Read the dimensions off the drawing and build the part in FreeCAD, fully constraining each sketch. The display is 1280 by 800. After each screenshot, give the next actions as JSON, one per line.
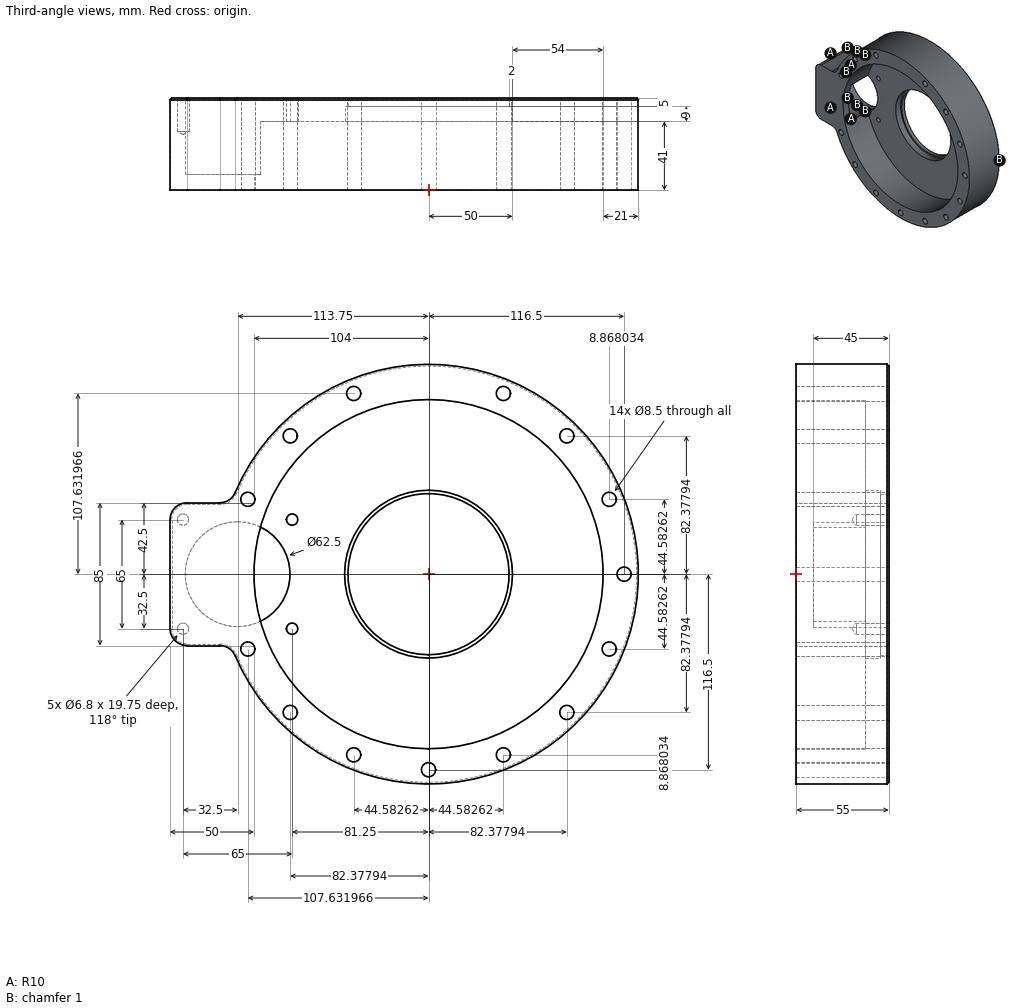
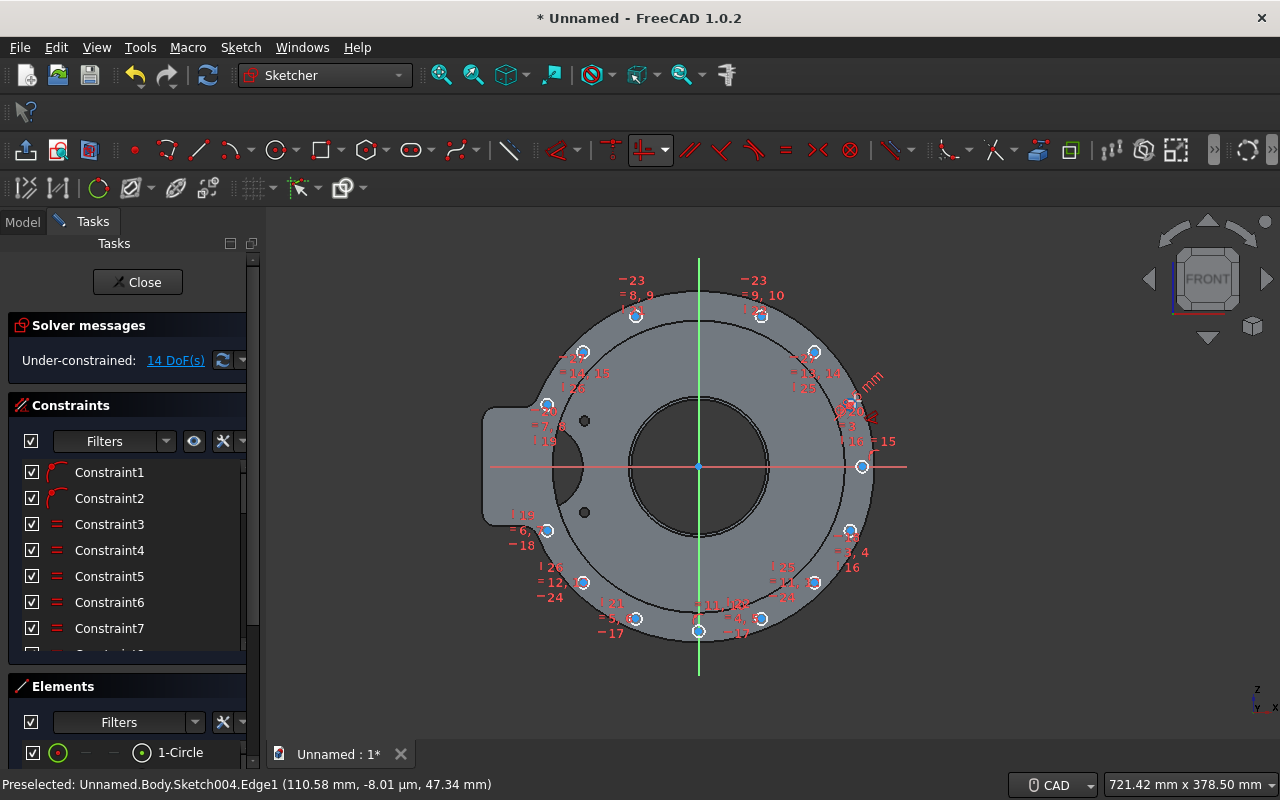
{"action": "left_click", "coordinate": [699, 631]}
{"action": "left_click", "coordinate": [665, 549]}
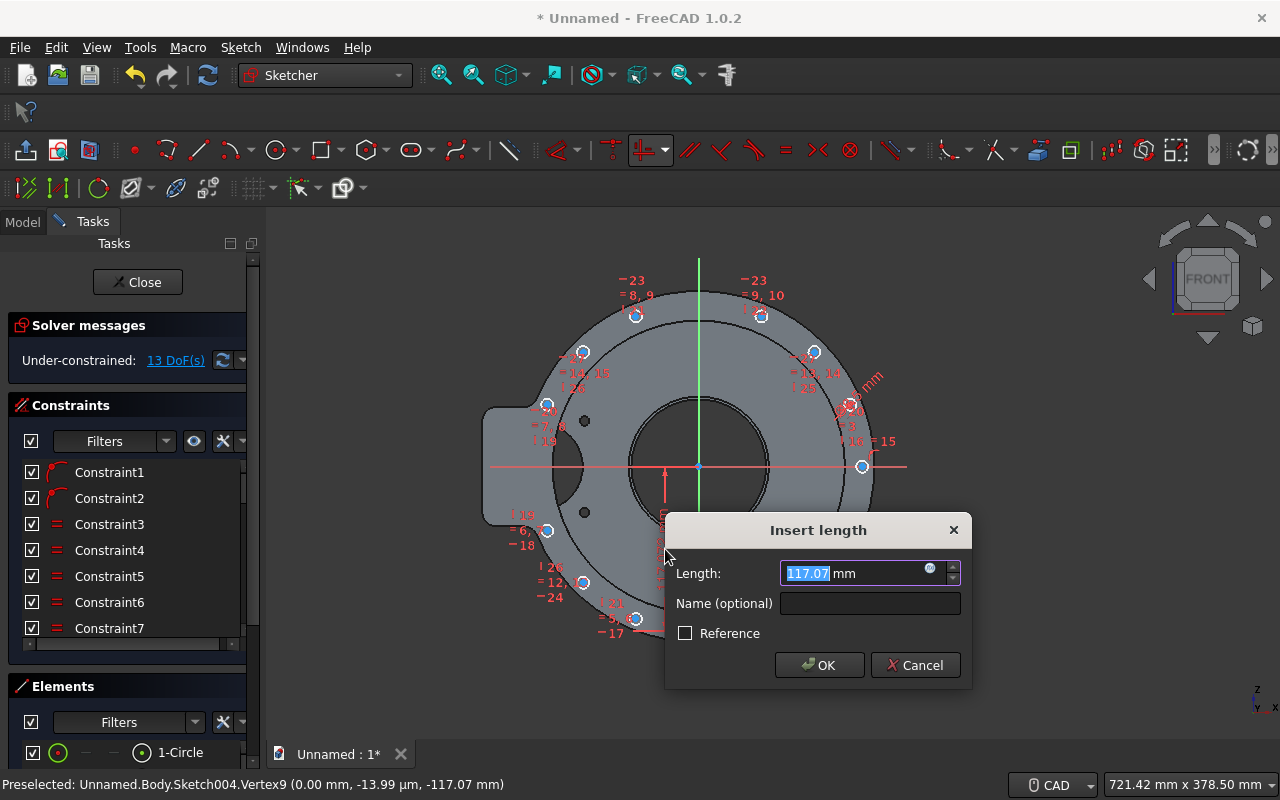
{"action": "type", "text": "116.5"}
{"action": "key", "text": "Return"}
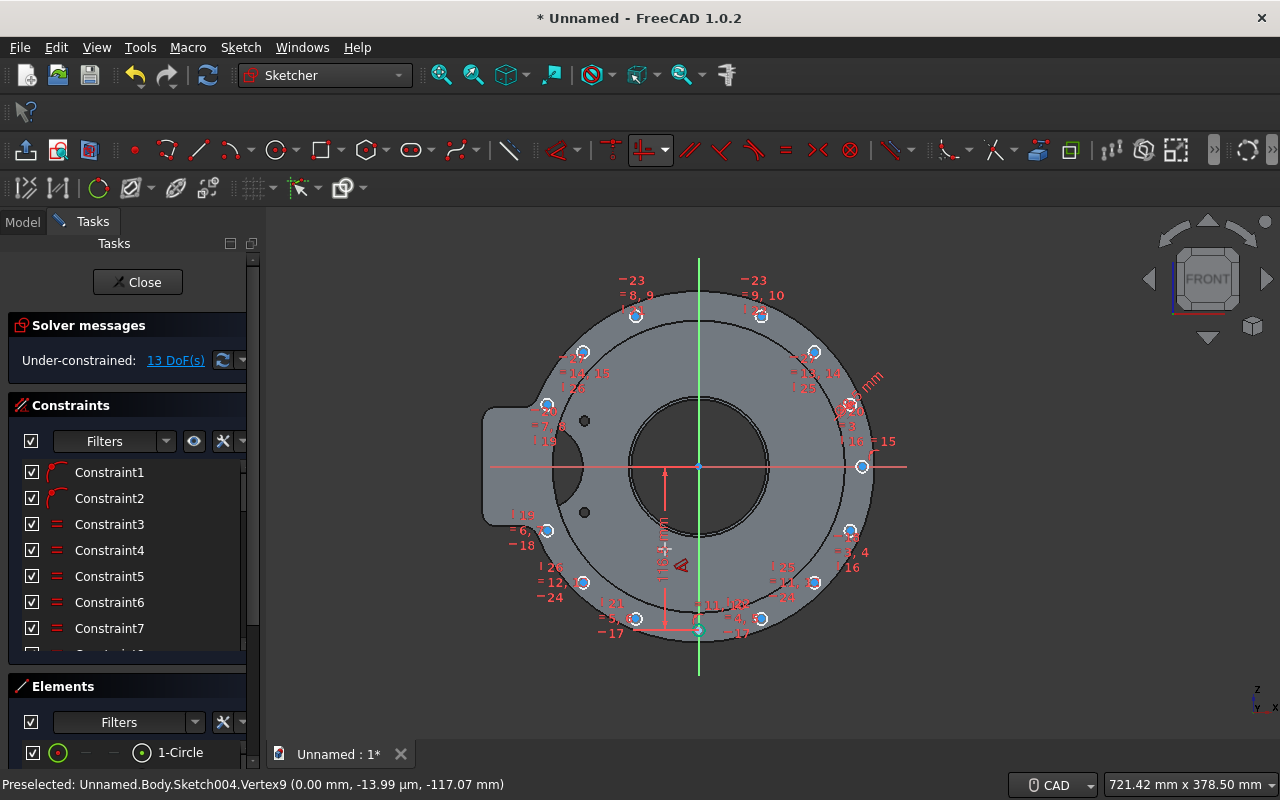
{"action": "left_click", "coordinate": [862, 467]}
{"action": "left_click", "coordinate": [780, 433]}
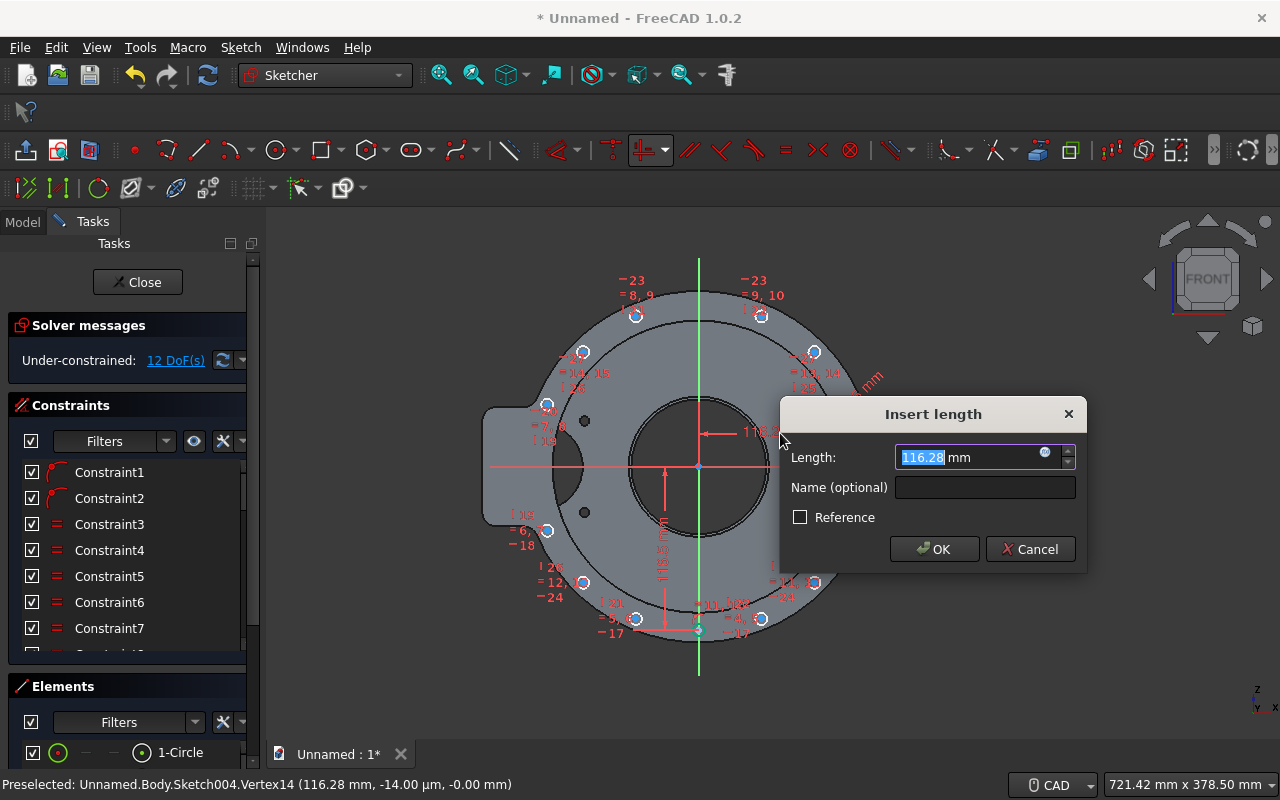
{"action": "type", "text": "116.5"}
{"action": "key", "text": "Return"}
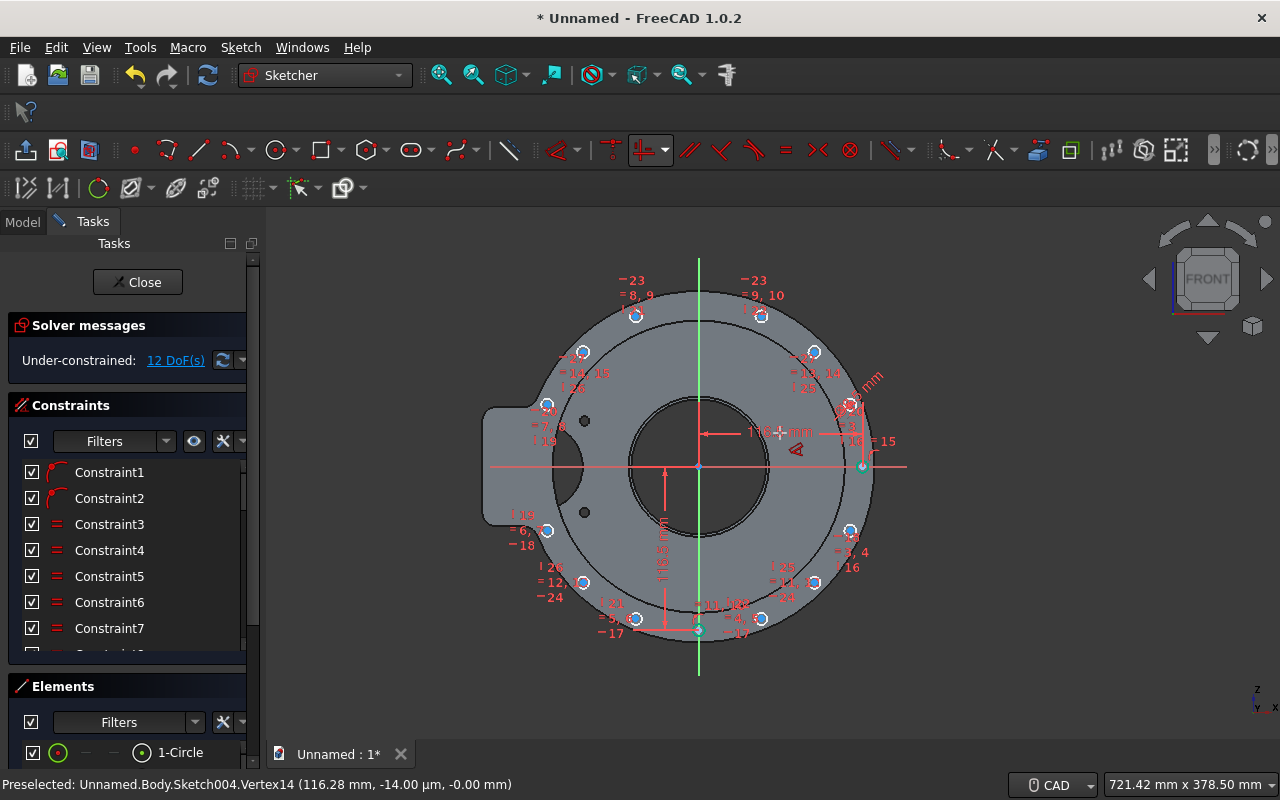
{"action": "left_click", "coordinate": [850, 405]}
{"action": "left_click", "coordinate": [884, 436]}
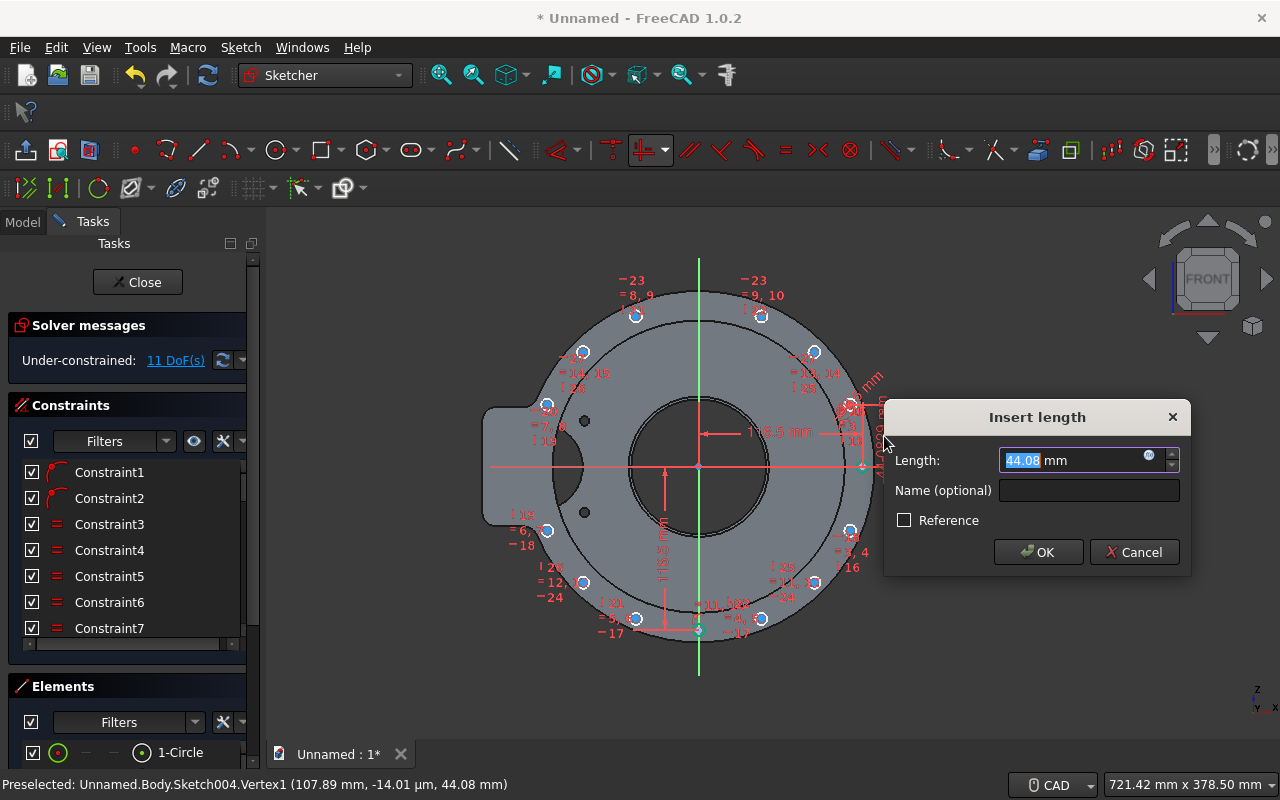
{"action": "type", "text": "44.58262"}
{"action": "key", "text": "Return"}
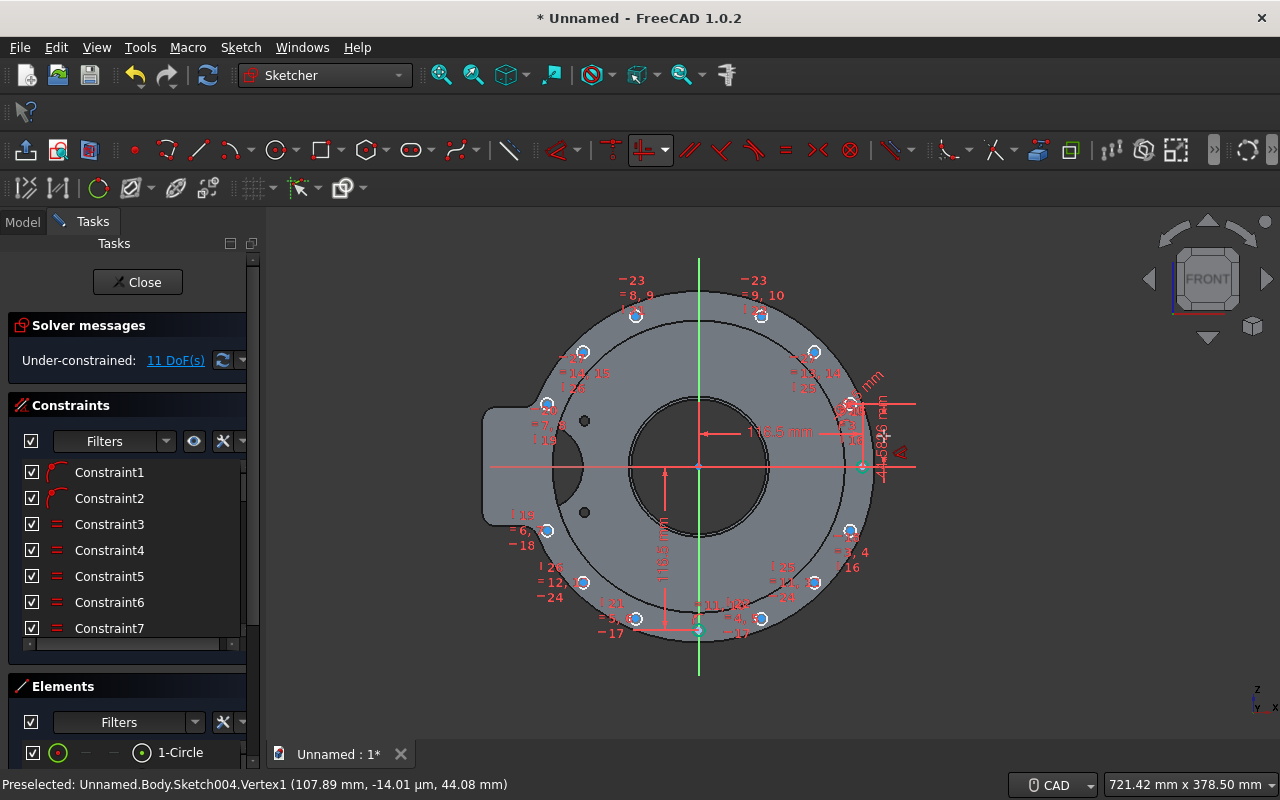
{"action": "left_click", "coordinate": [850, 531]}
{"action": "left_click", "coordinate": [884, 499]}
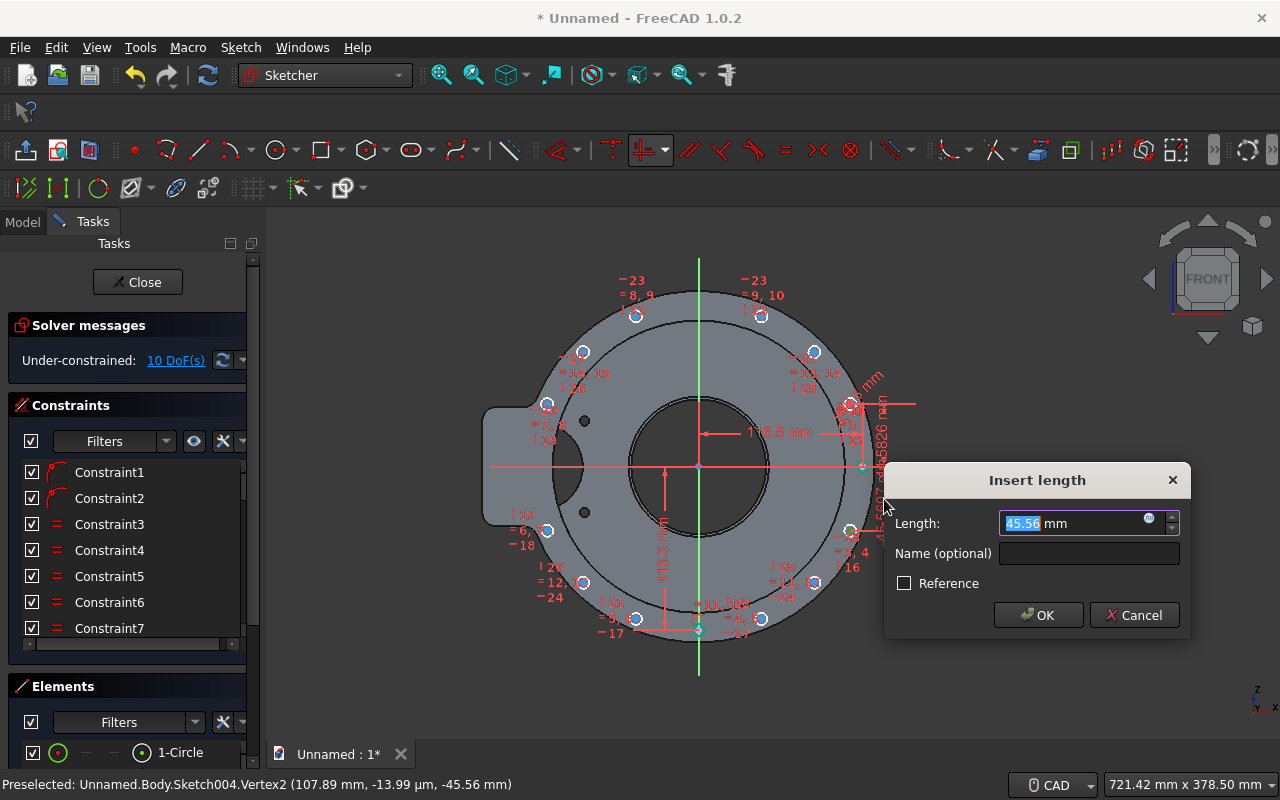
{"action": "type", "text": "44.58262"}
{"action": "key", "text": "Return"}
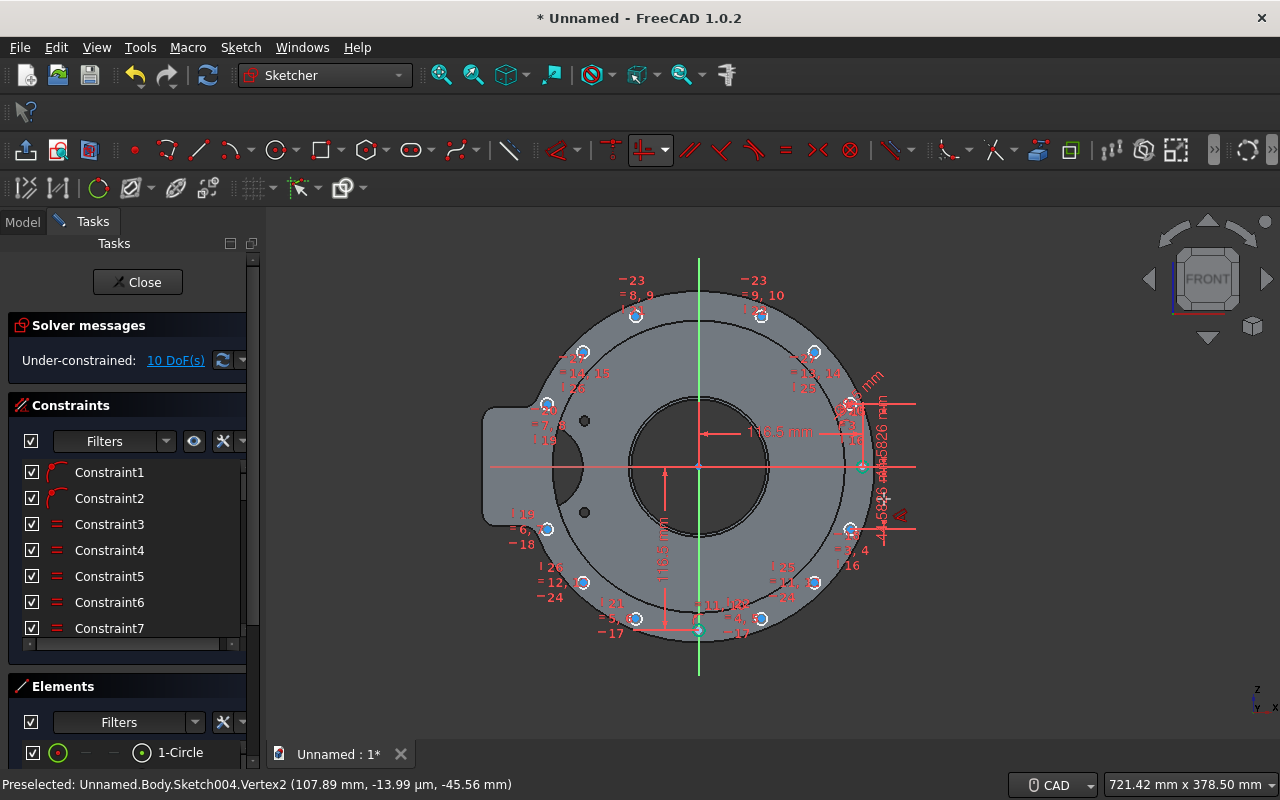
{"action": "left_click", "coordinate": [761, 619]}
{"action": "left_click", "coordinate": [730, 653]}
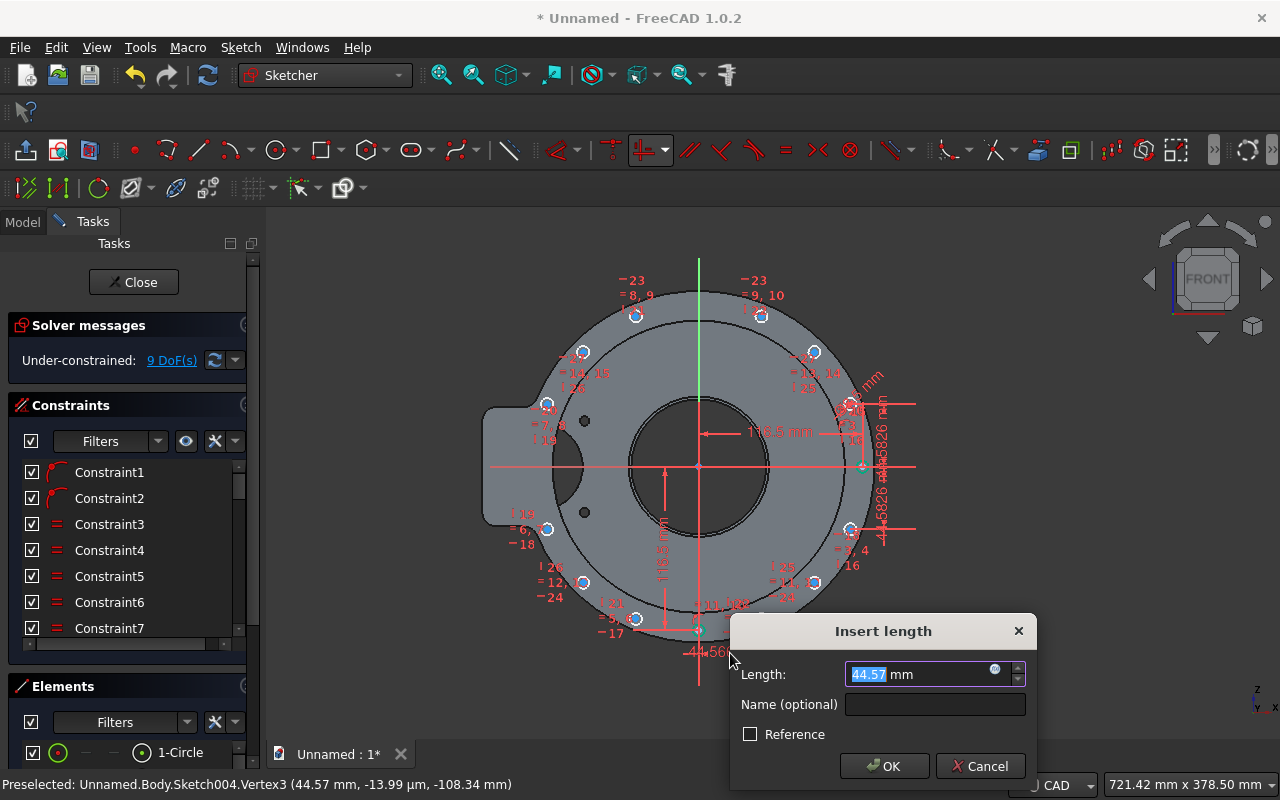
{"action": "type", "text": "44.58262"}
{"action": "key", "text": "Return"}